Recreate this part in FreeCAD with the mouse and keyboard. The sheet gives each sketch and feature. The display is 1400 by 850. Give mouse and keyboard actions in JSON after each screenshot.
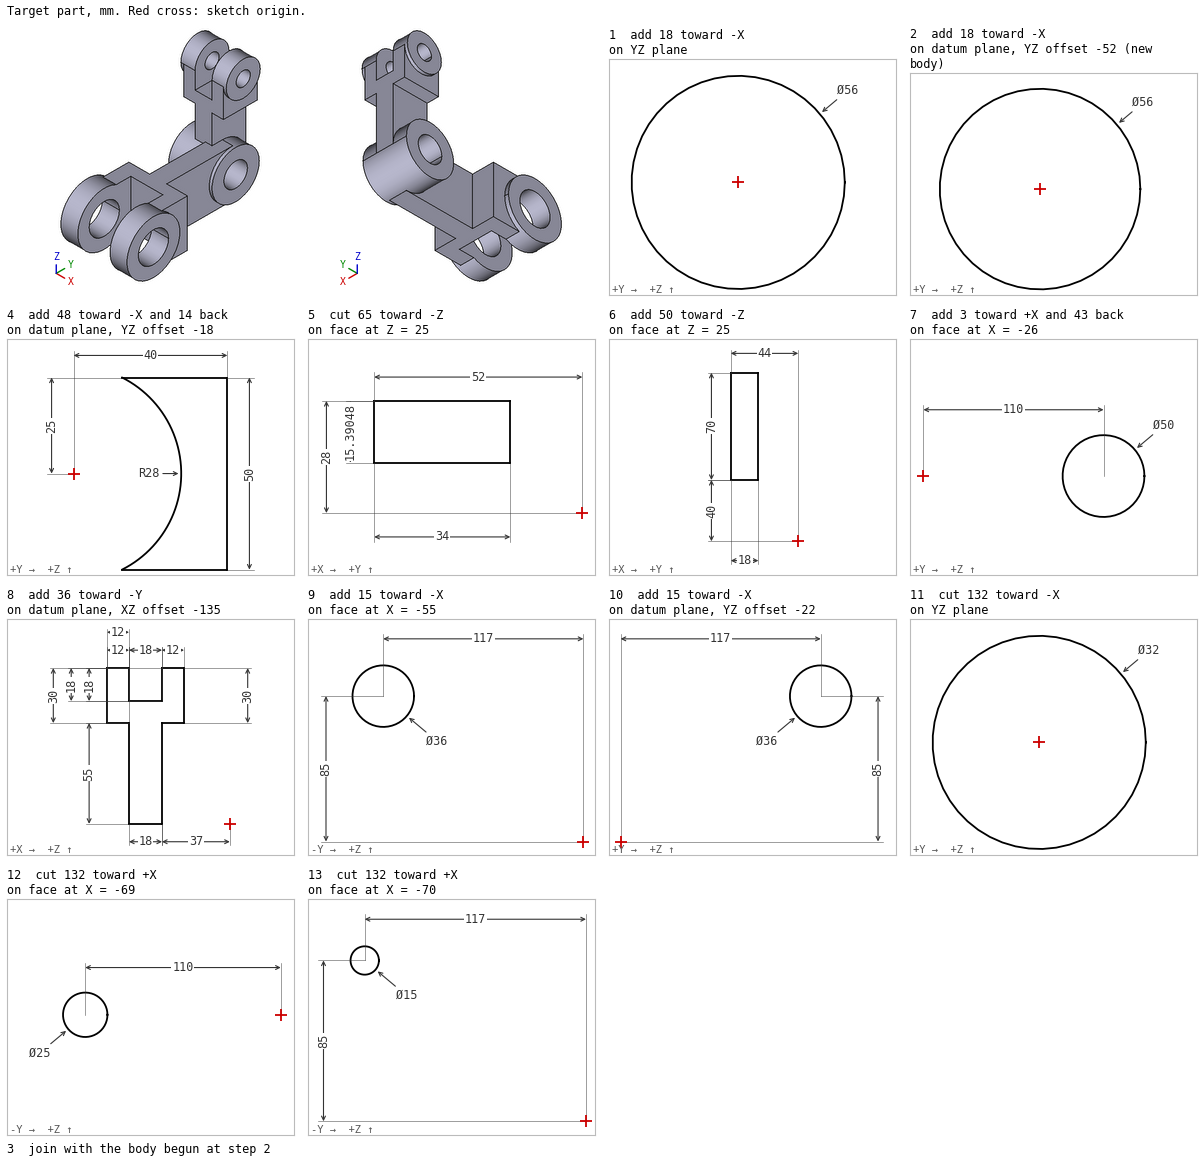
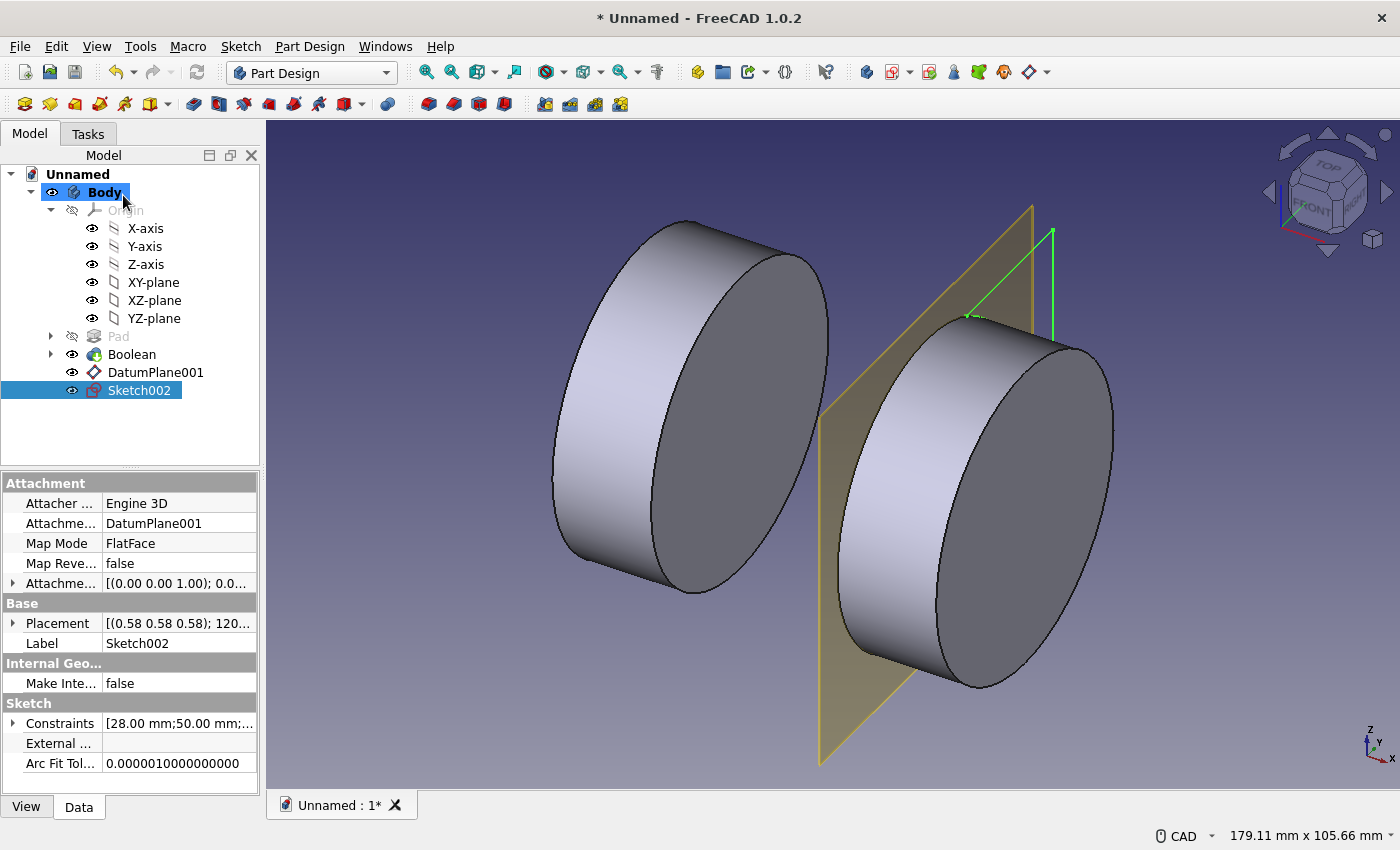
{"action": "left_click", "coordinate": [25, 104]}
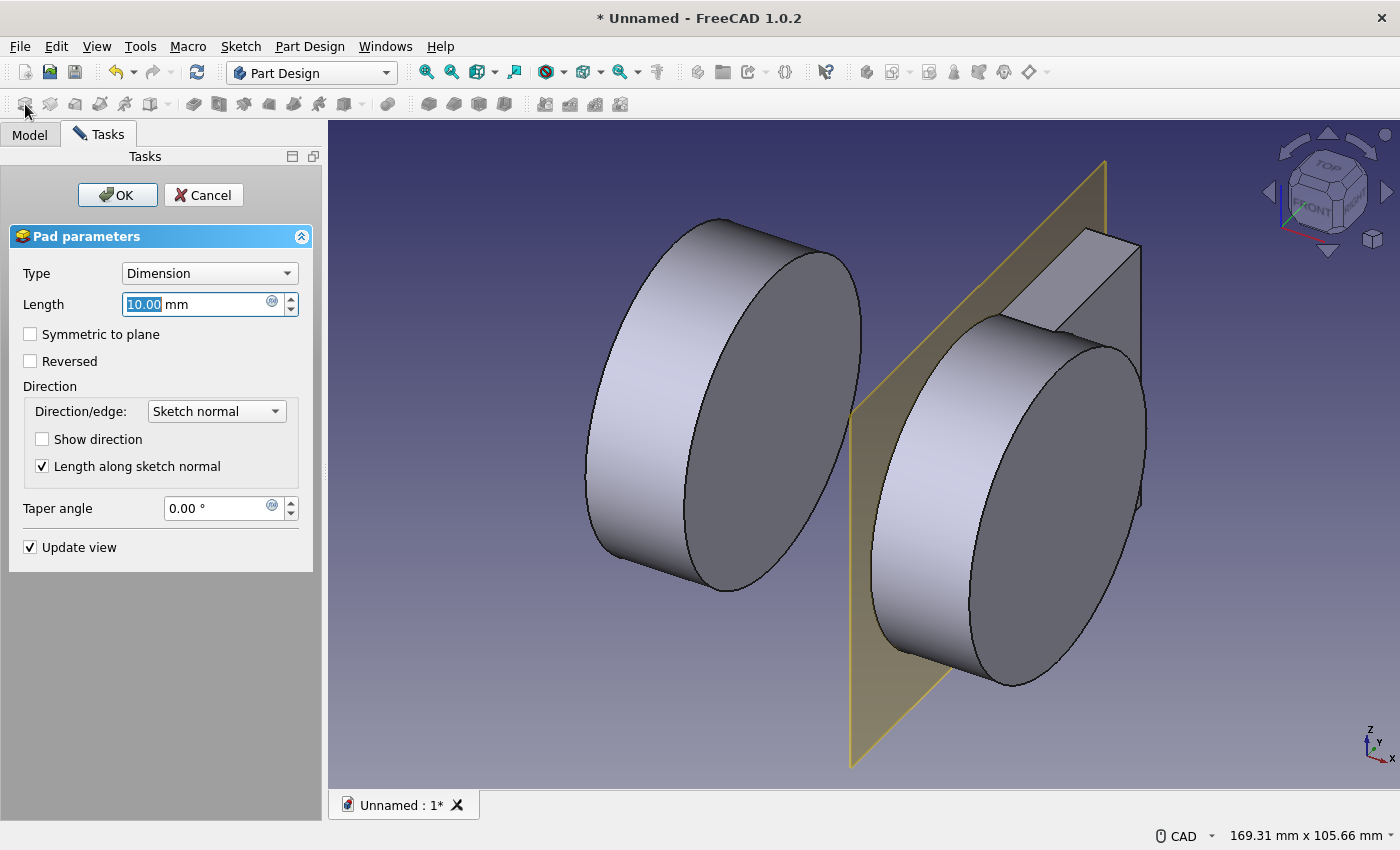
{"action": "left_click", "coordinate": [210, 274]}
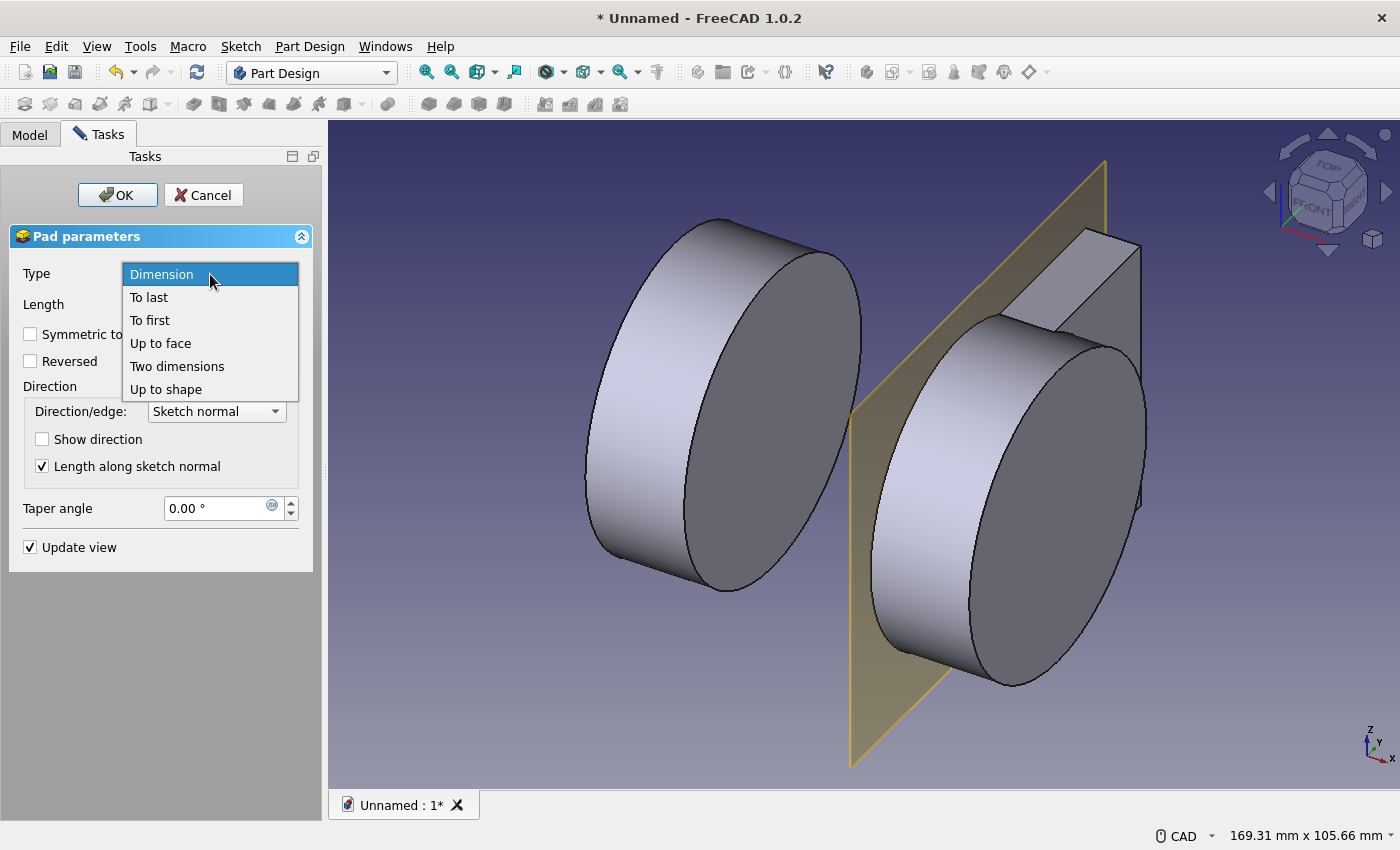
{"action": "left_click", "coordinate": [208, 366]}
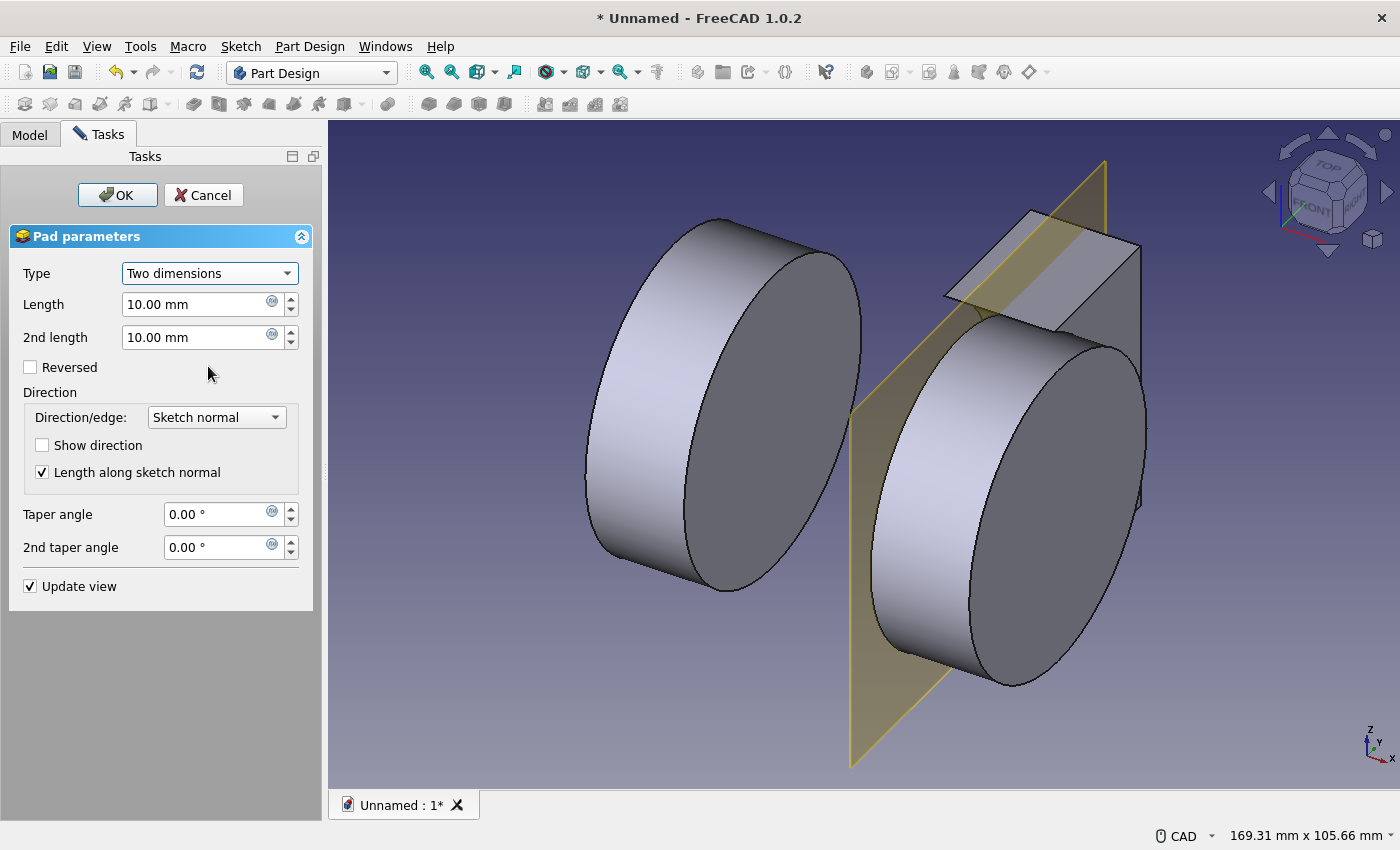
{"action": "triple_click", "coordinate": [204, 304]}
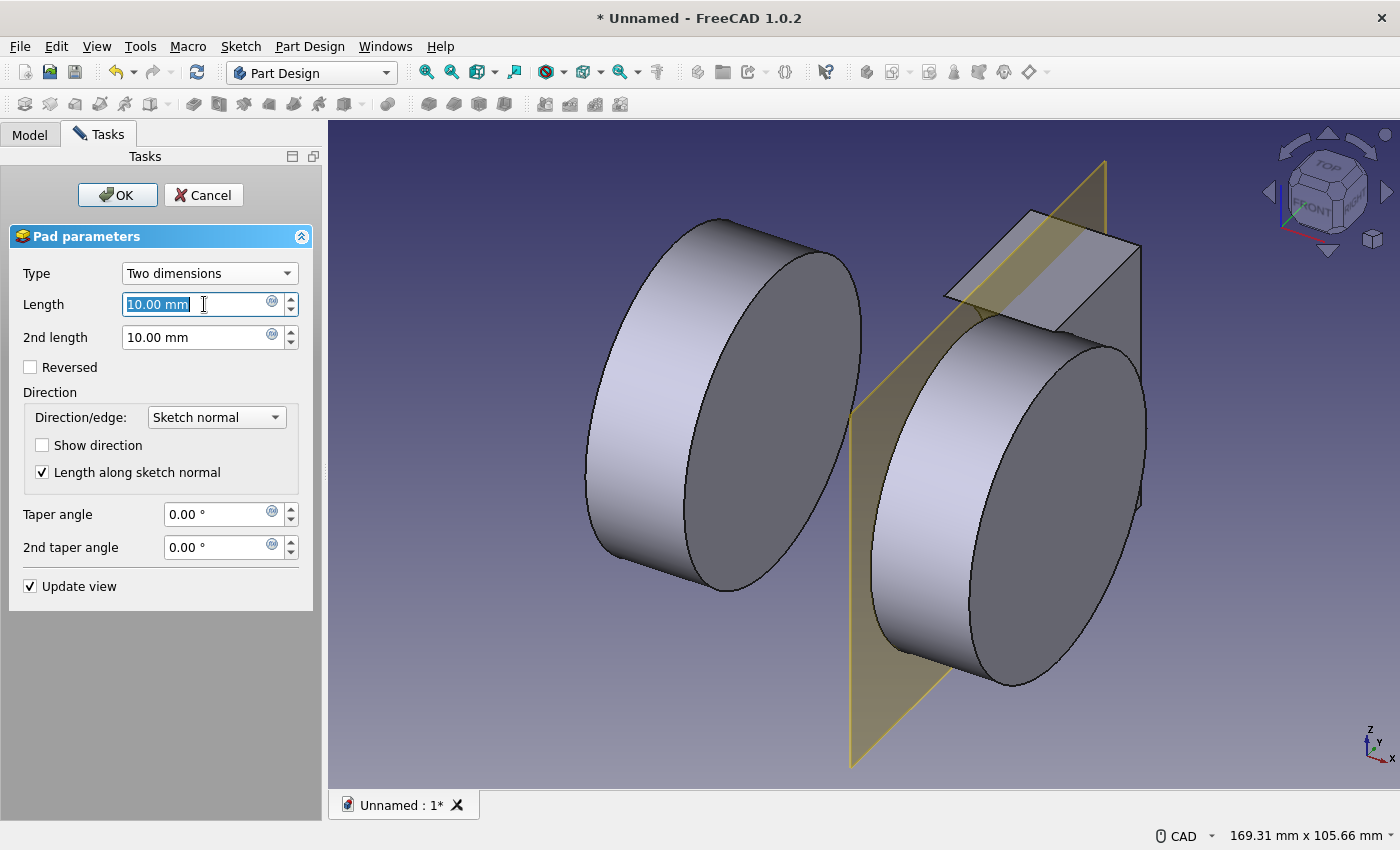
{"action": "type", "text": "48"}
{"action": "key", "text": "Tab"}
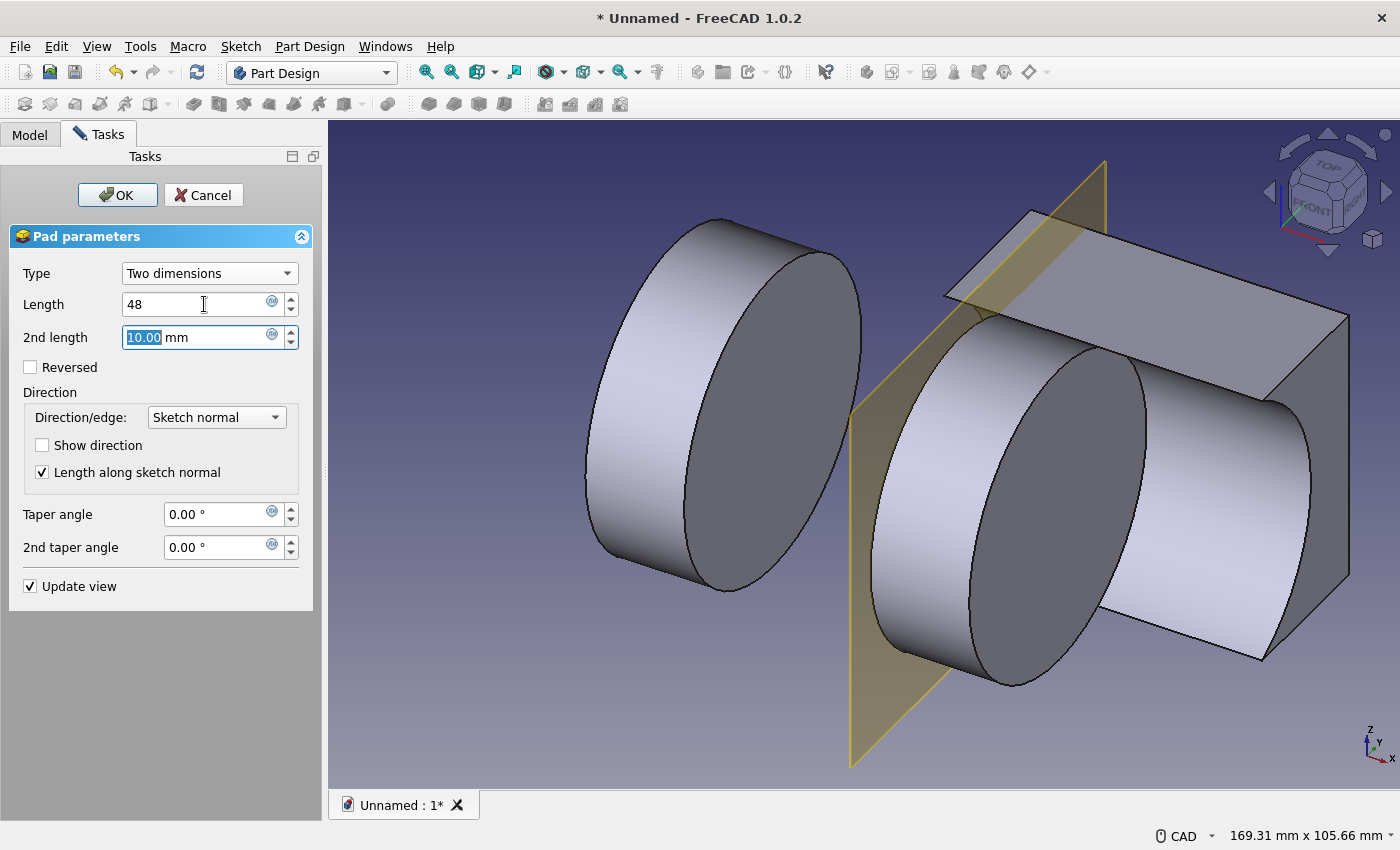
{"action": "type", "text": "14"}
{"action": "key", "text": "Tab"}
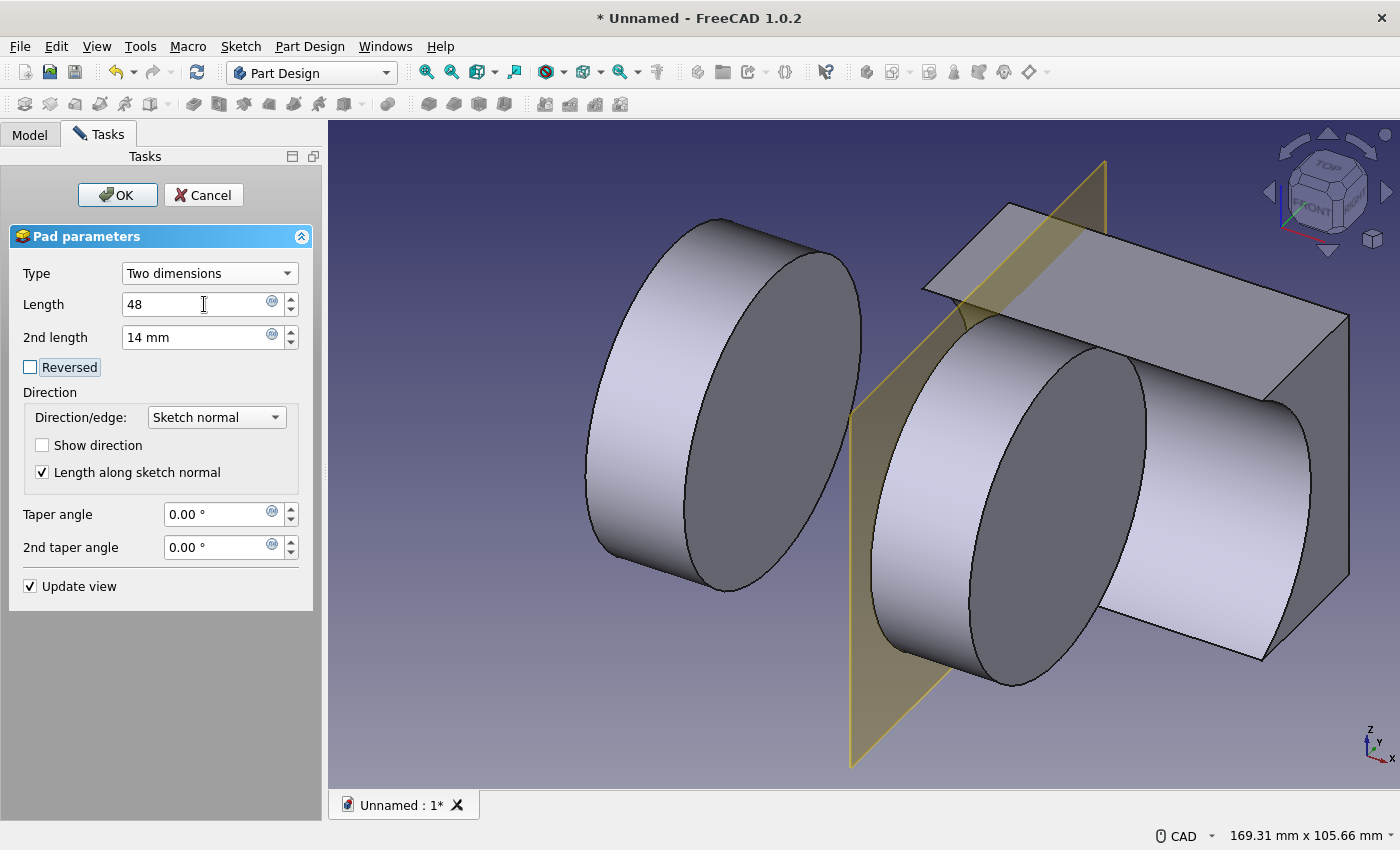
{"action": "left_click", "coordinate": [31, 367]}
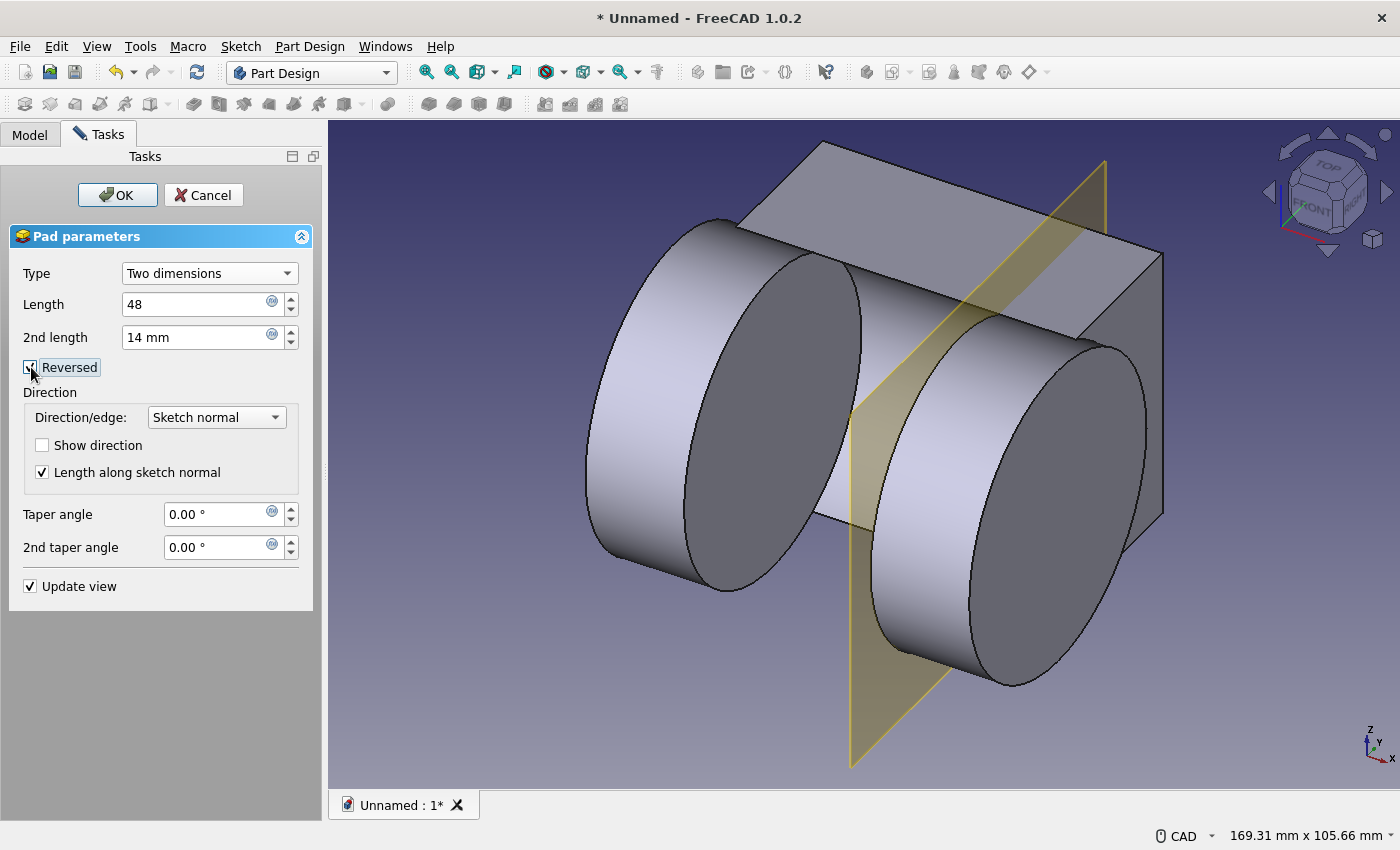
{"action": "left_click", "coordinate": [118, 195]}